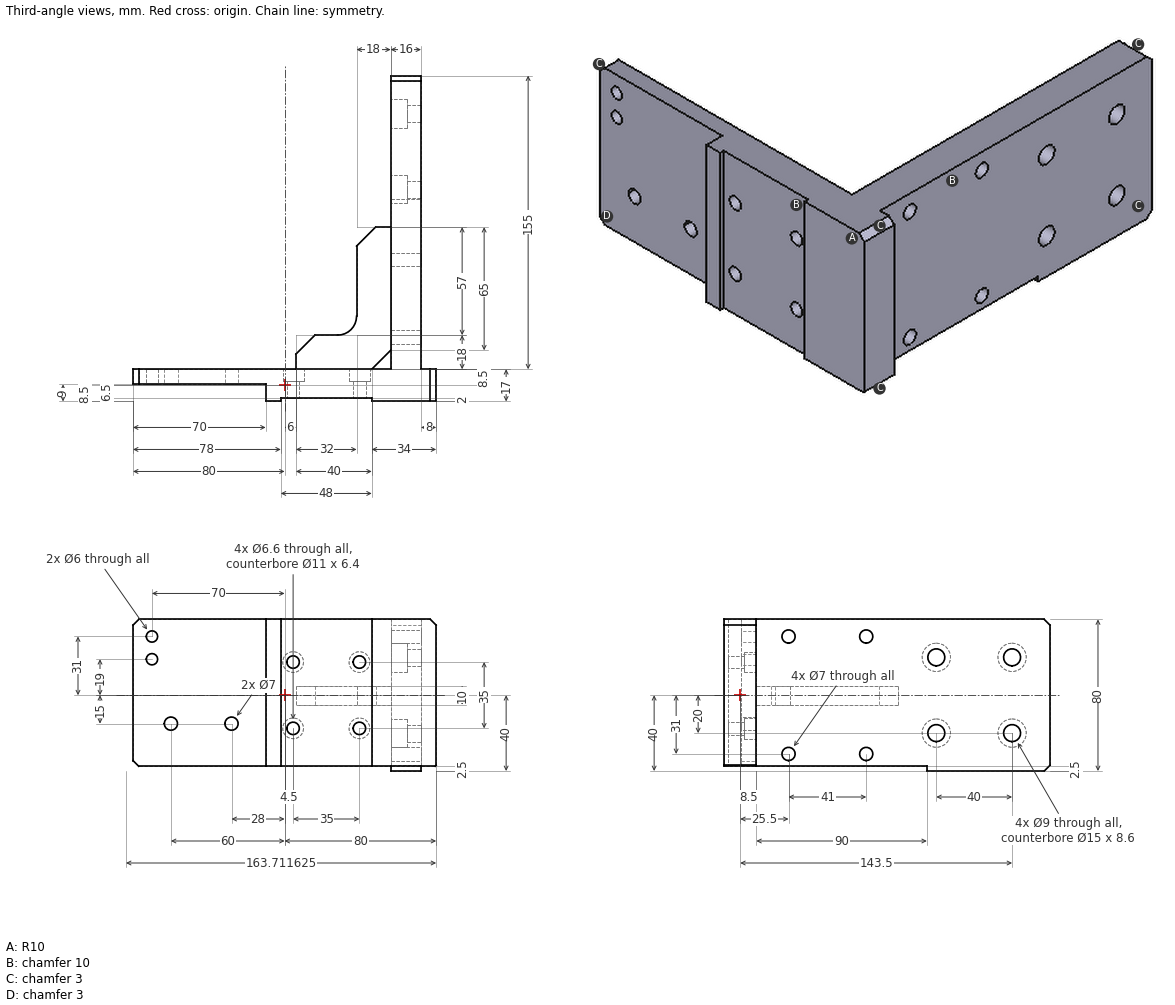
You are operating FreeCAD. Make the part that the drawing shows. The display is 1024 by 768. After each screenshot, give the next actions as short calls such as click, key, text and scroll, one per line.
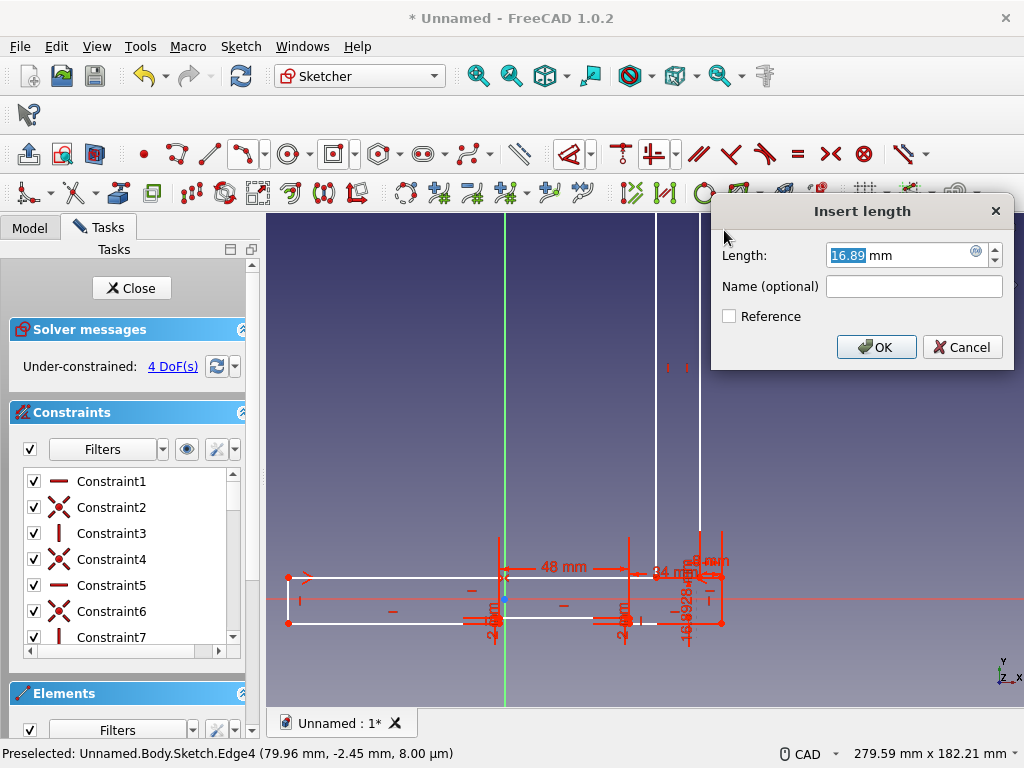
text(17)
key(Return)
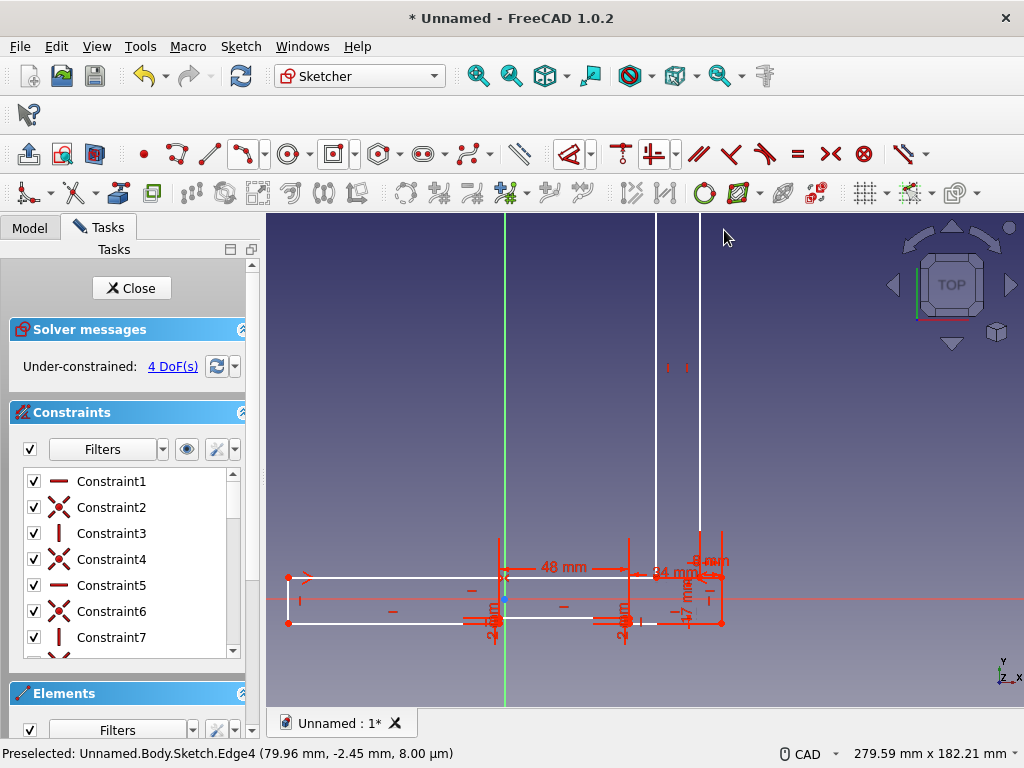
scroll(722, 604, down, 2)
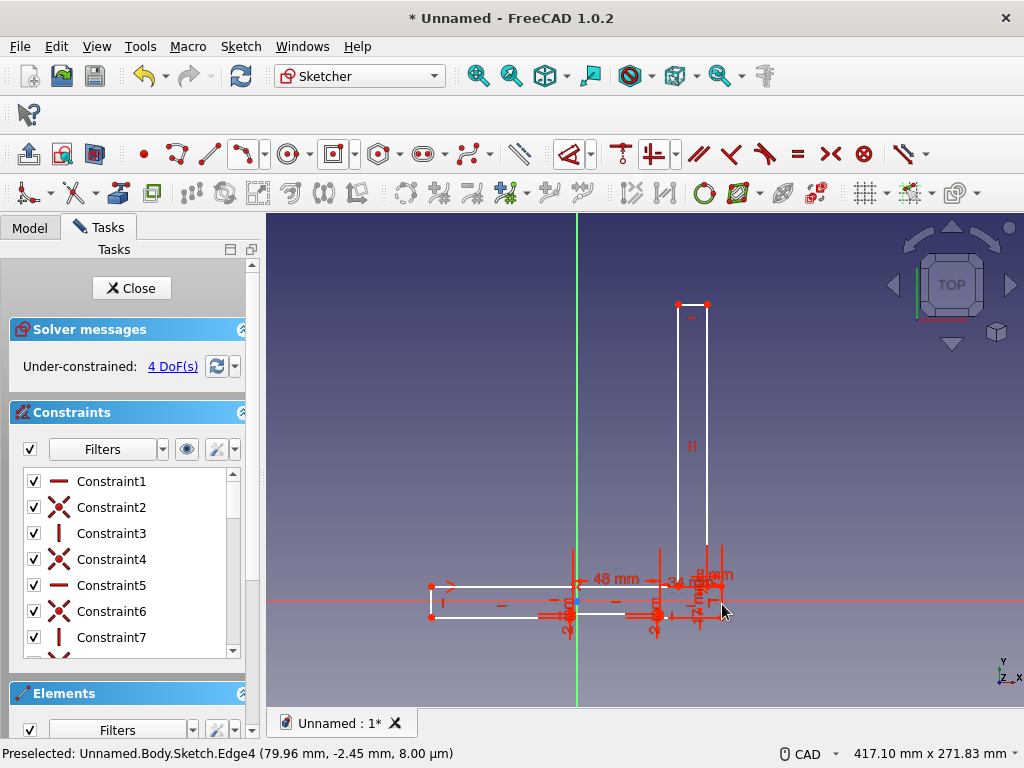
scroll(699, 305, up, 3)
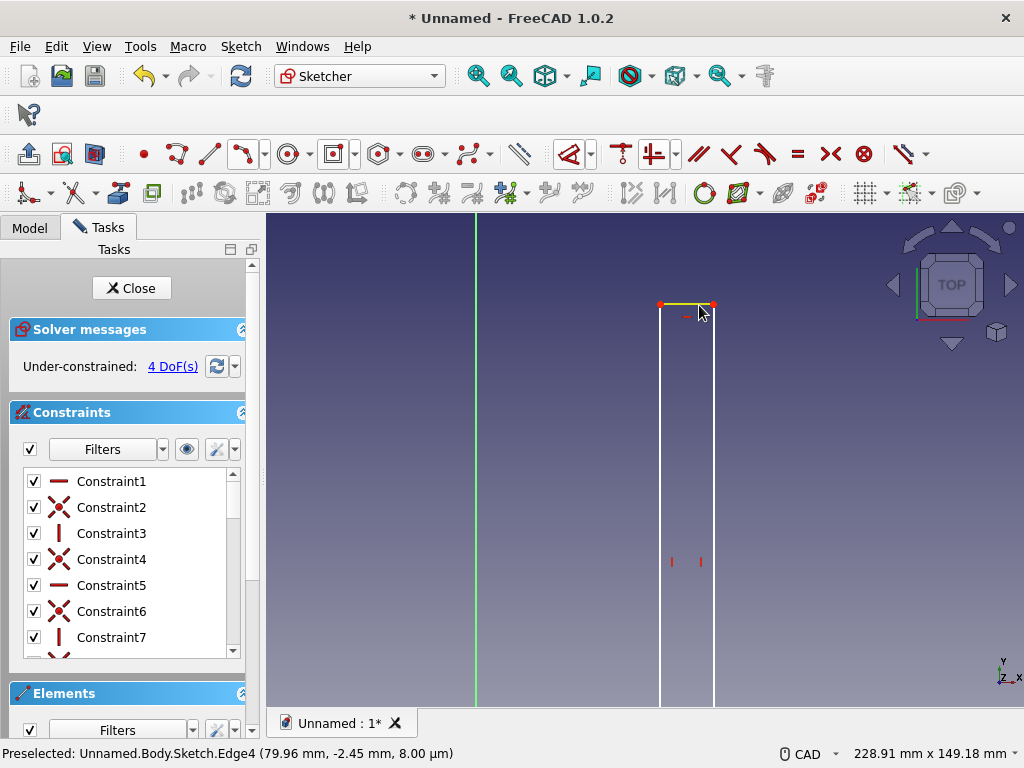
click(698, 304)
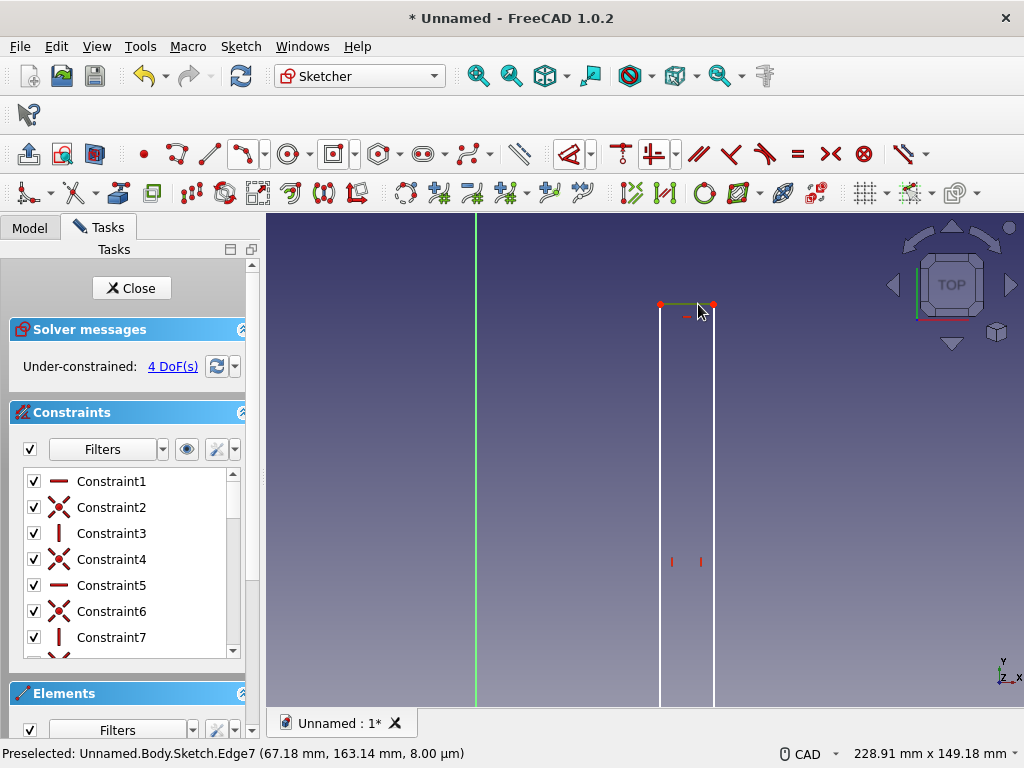
click(590, 154)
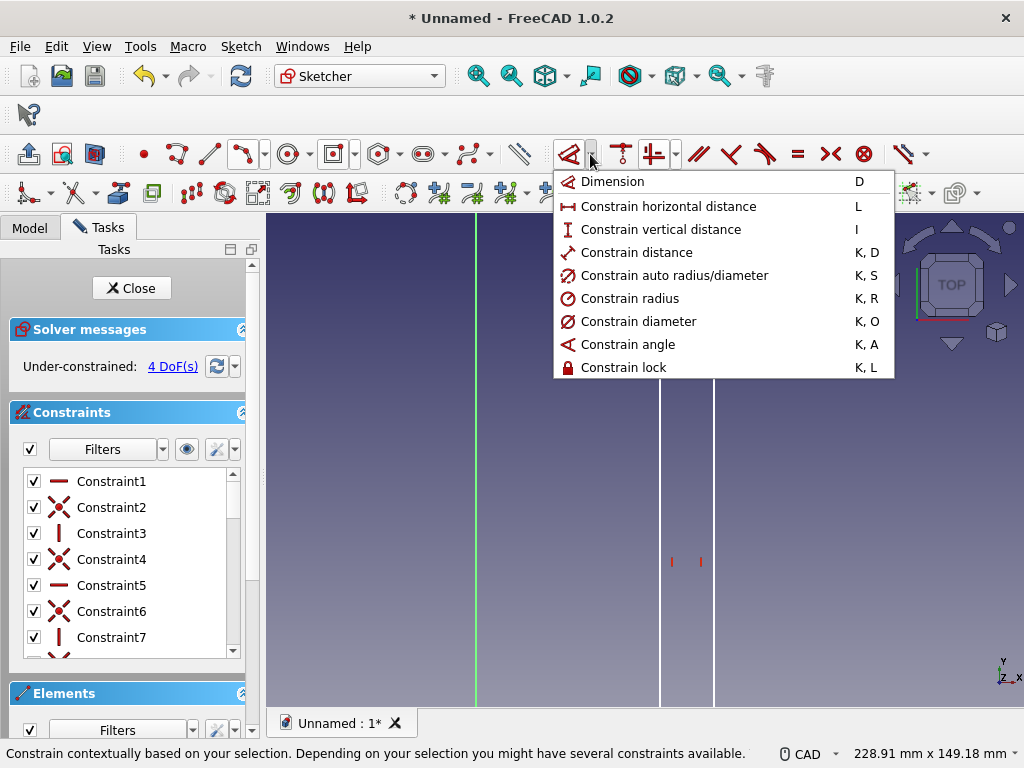
click(724, 206)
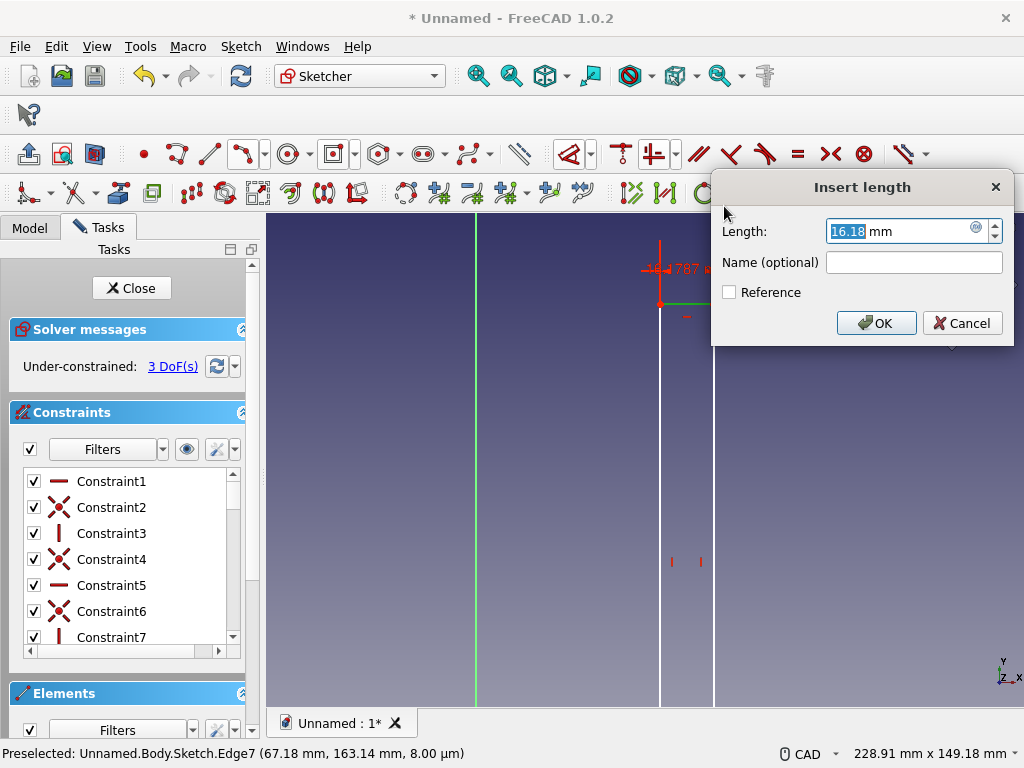
text(16)
key(Return)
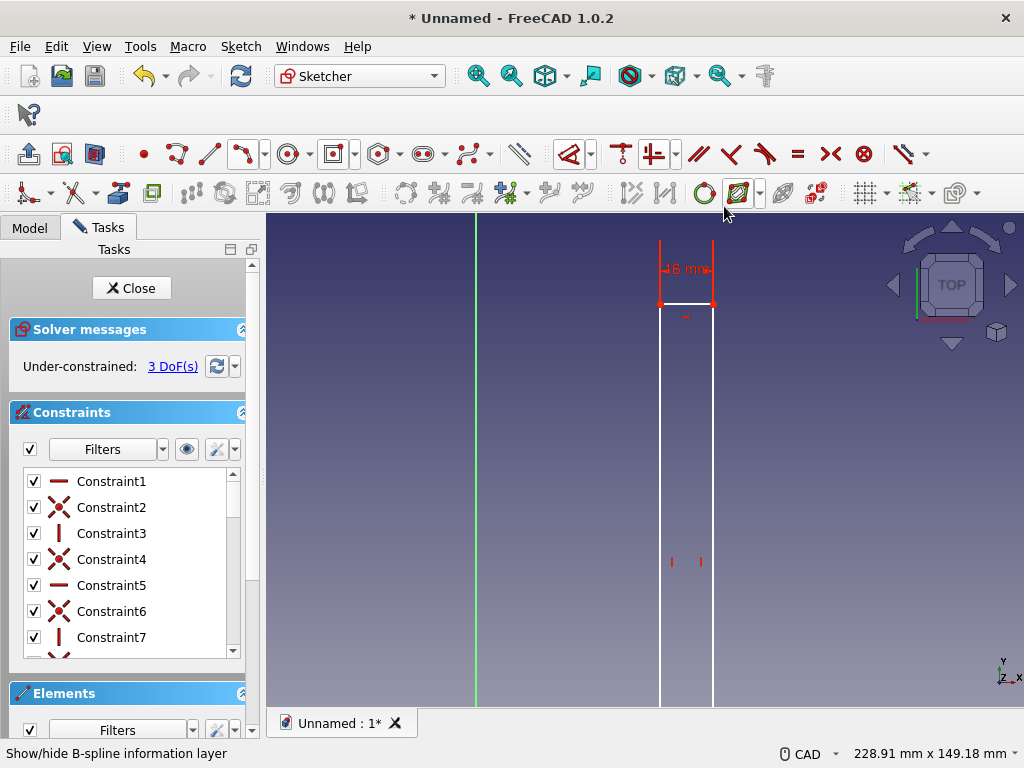
scroll(699, 304, down, 3)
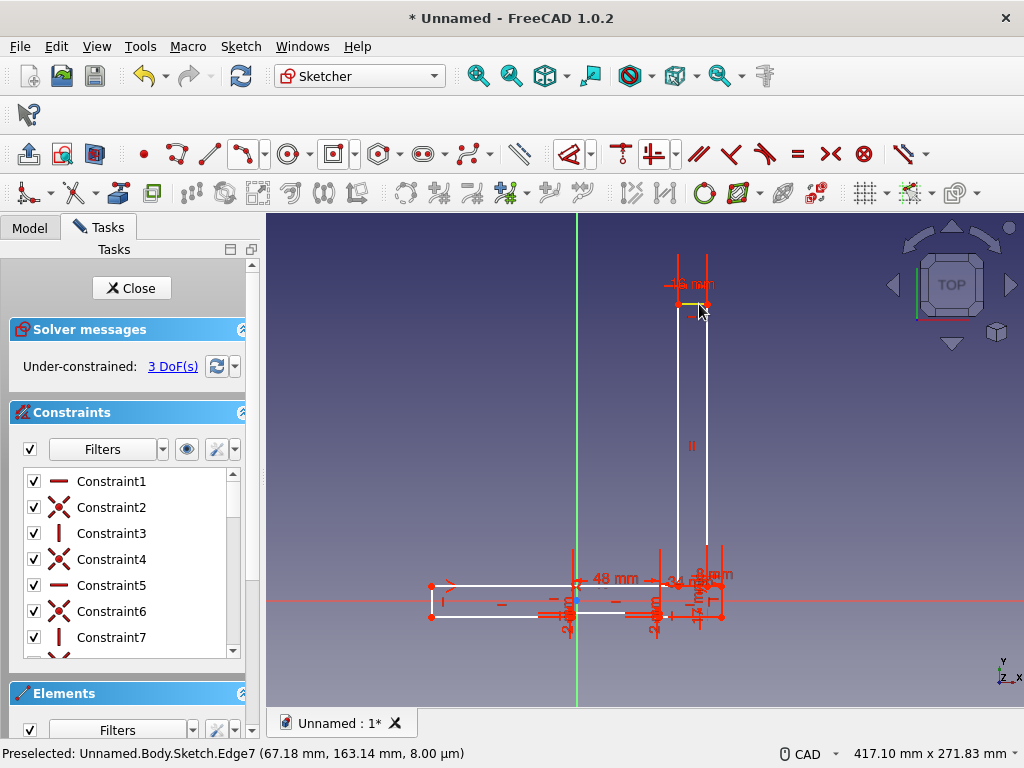
click(474, 617)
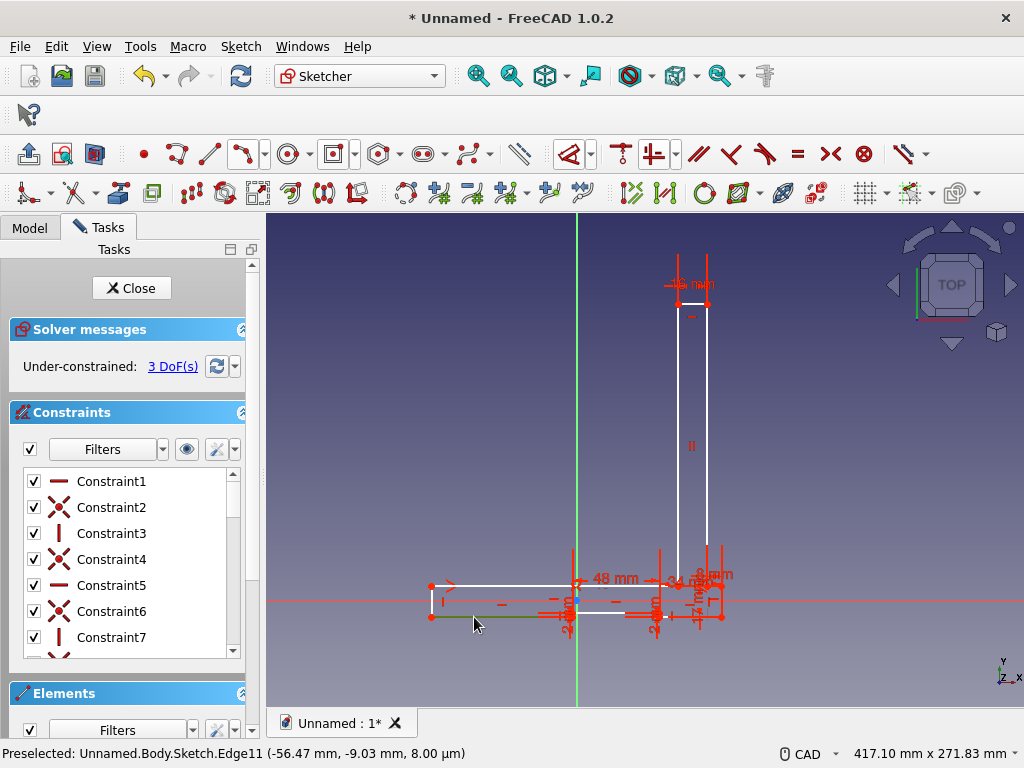
click(590, 154)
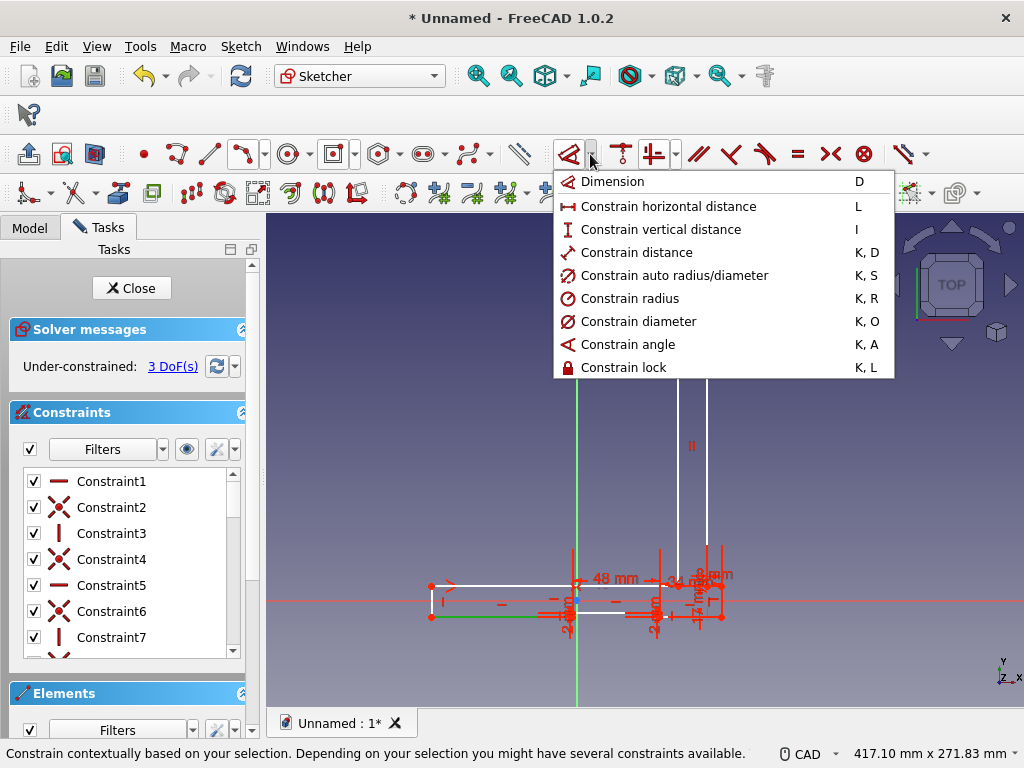
click(724, 206)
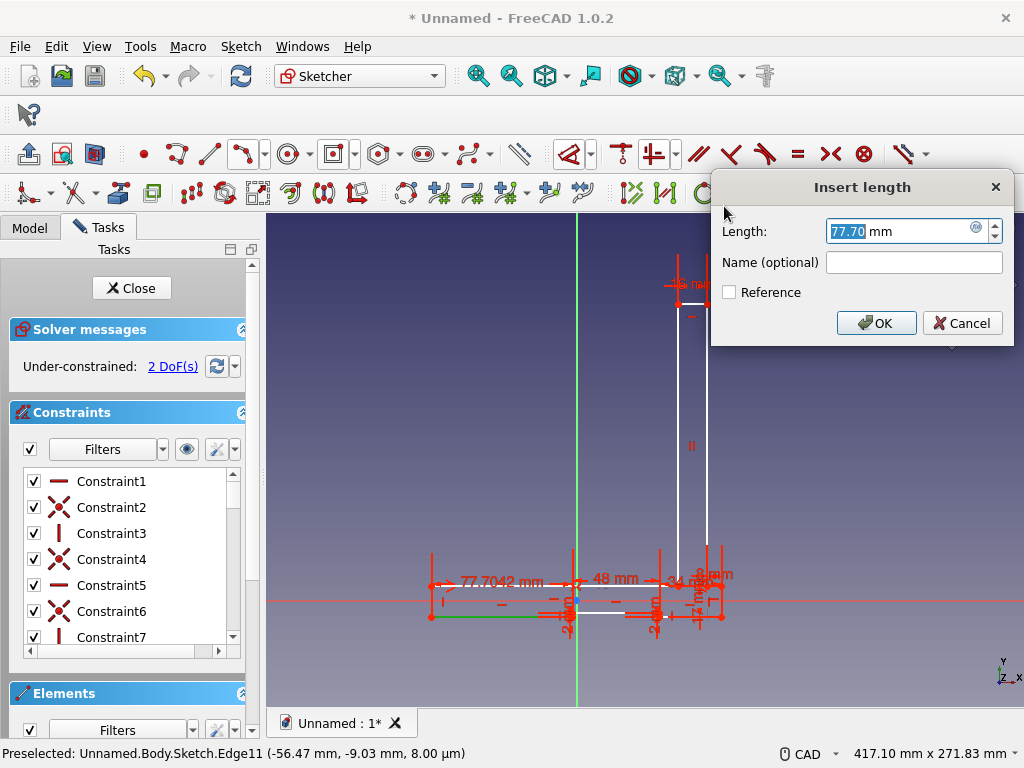
text(78)
key(Return)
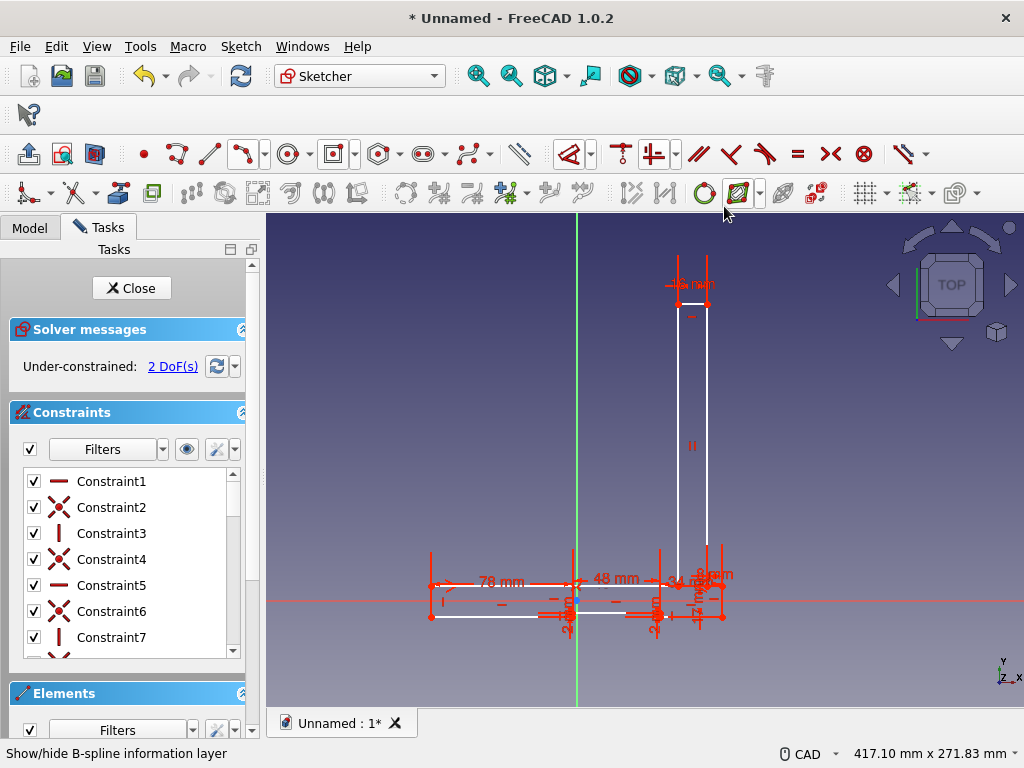
click(707, 502)